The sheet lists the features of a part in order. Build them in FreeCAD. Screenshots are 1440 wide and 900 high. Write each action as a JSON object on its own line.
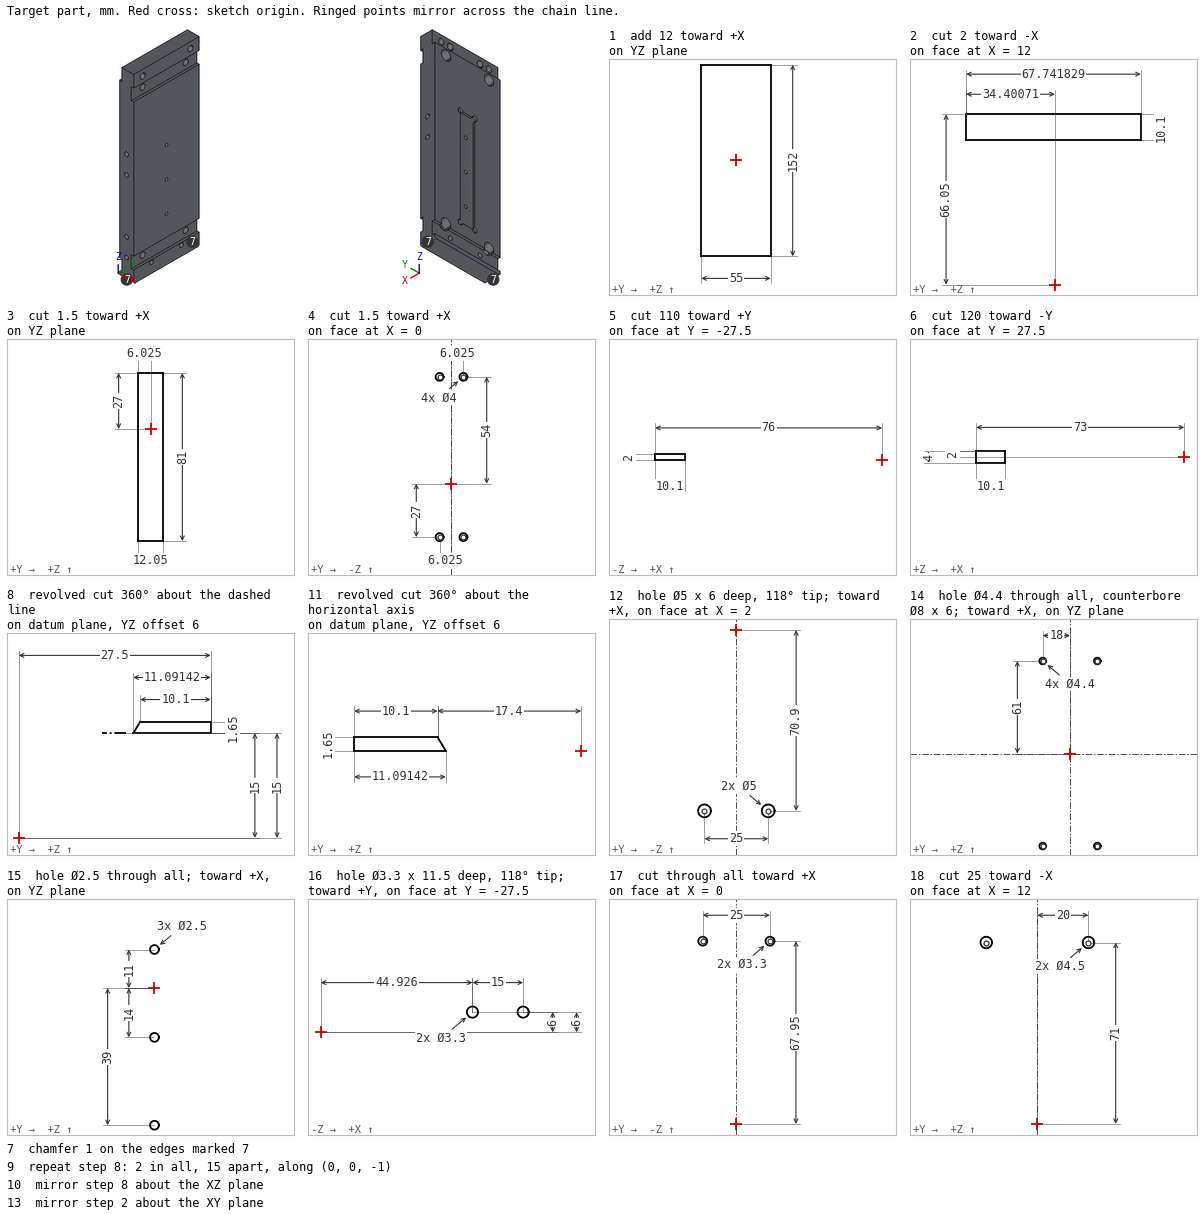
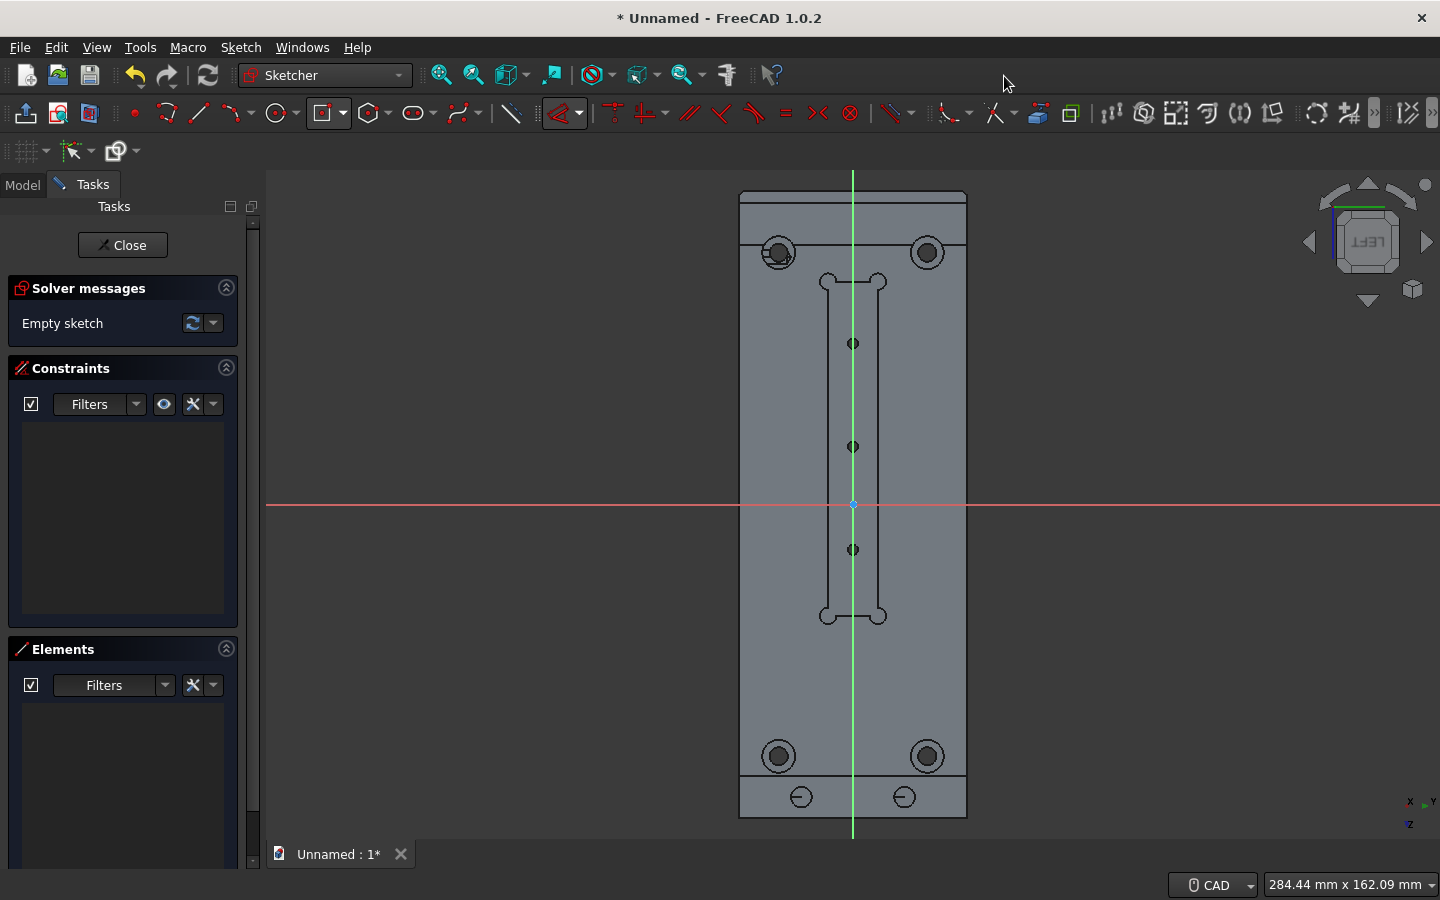
{"action": "scroll", "coordinate": [992, 198], "scroll_direction": "up", "scroll_amount": 2}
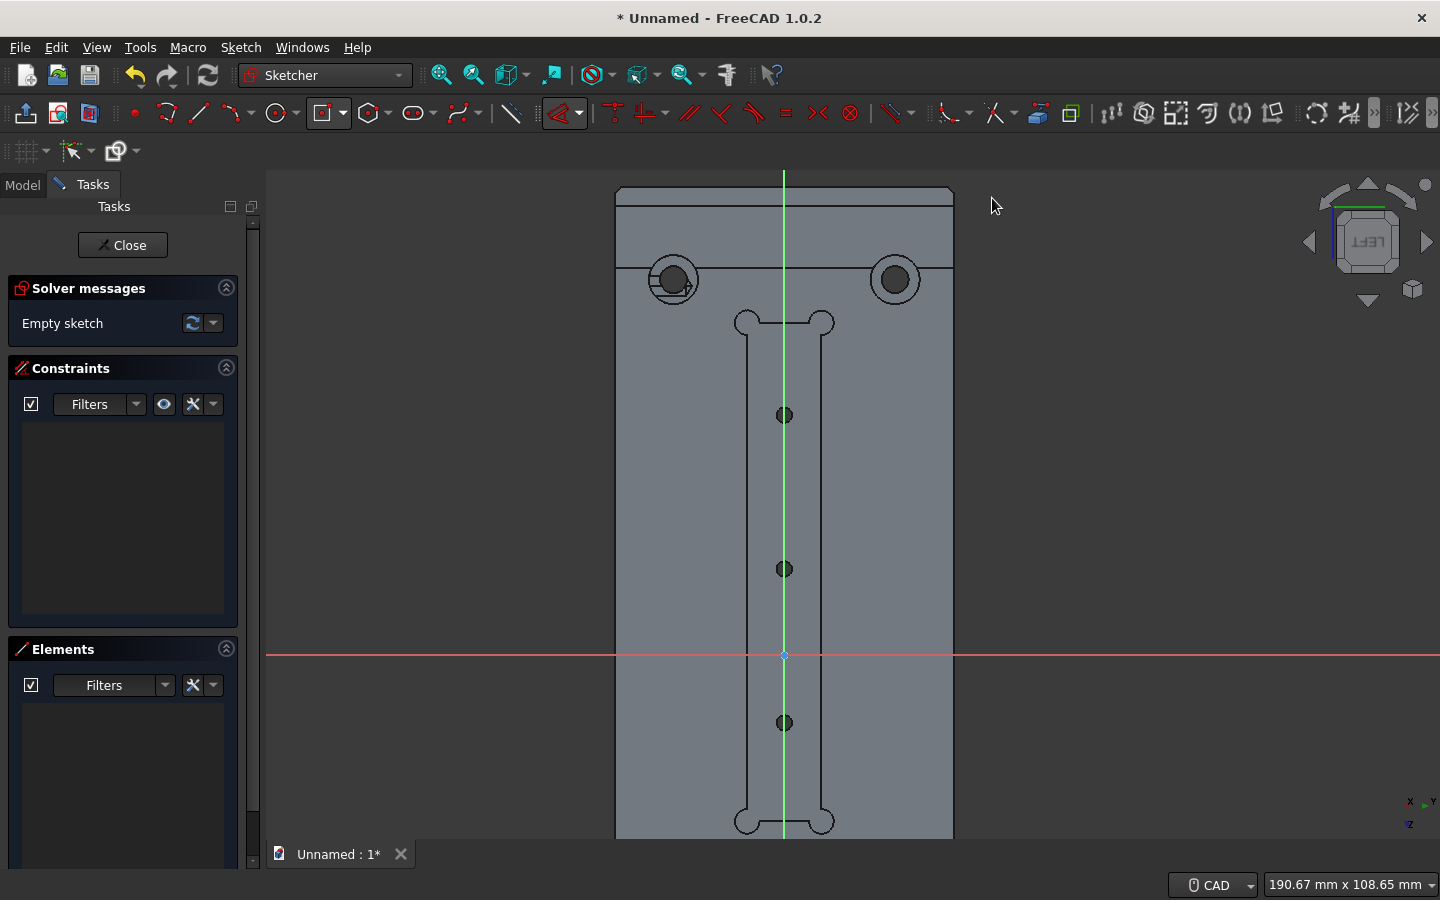
{"action": "left_click", "coordinate": [276, 114]}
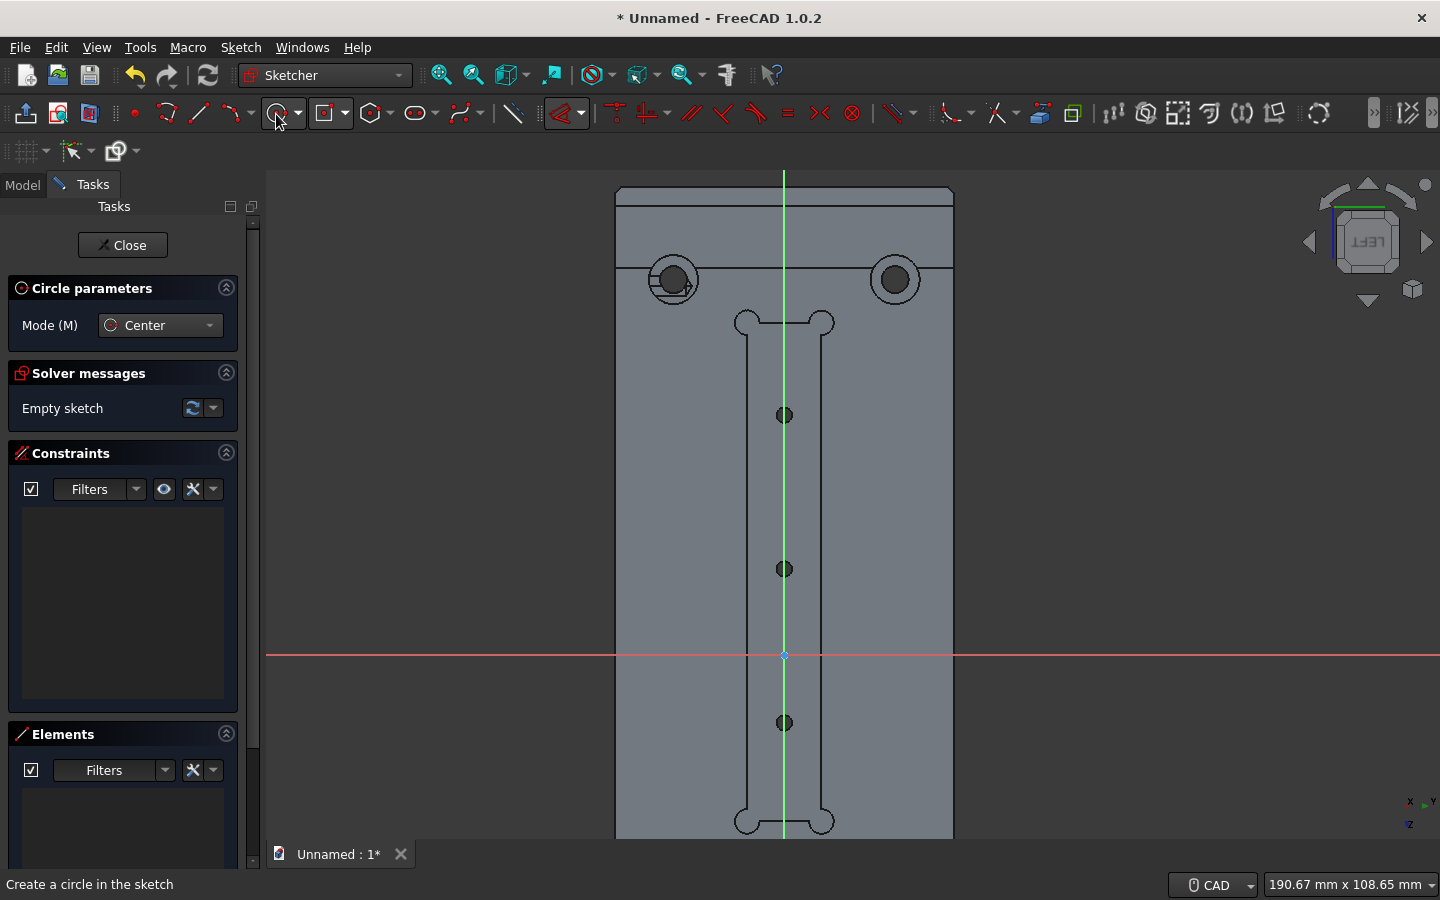
{"action": "scroll", "coordinate": [861, 237], "scroll_direction": "up", "scroll_amount": 5}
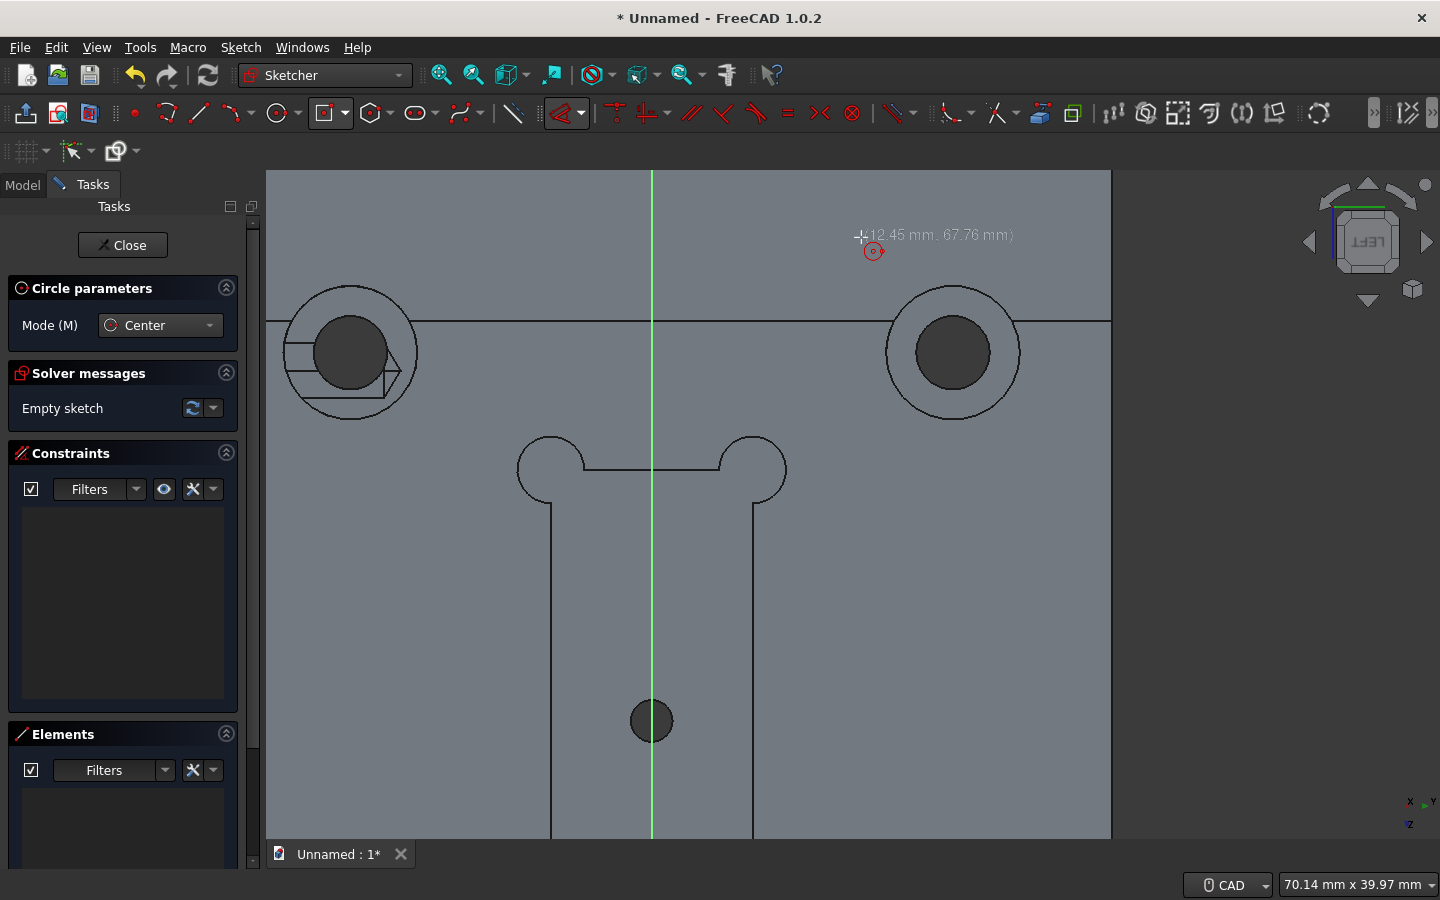
{"action": "left_click", "coordinate": [861, 236]}
{"action": "mouse_move", "coordinate": [880, 217]}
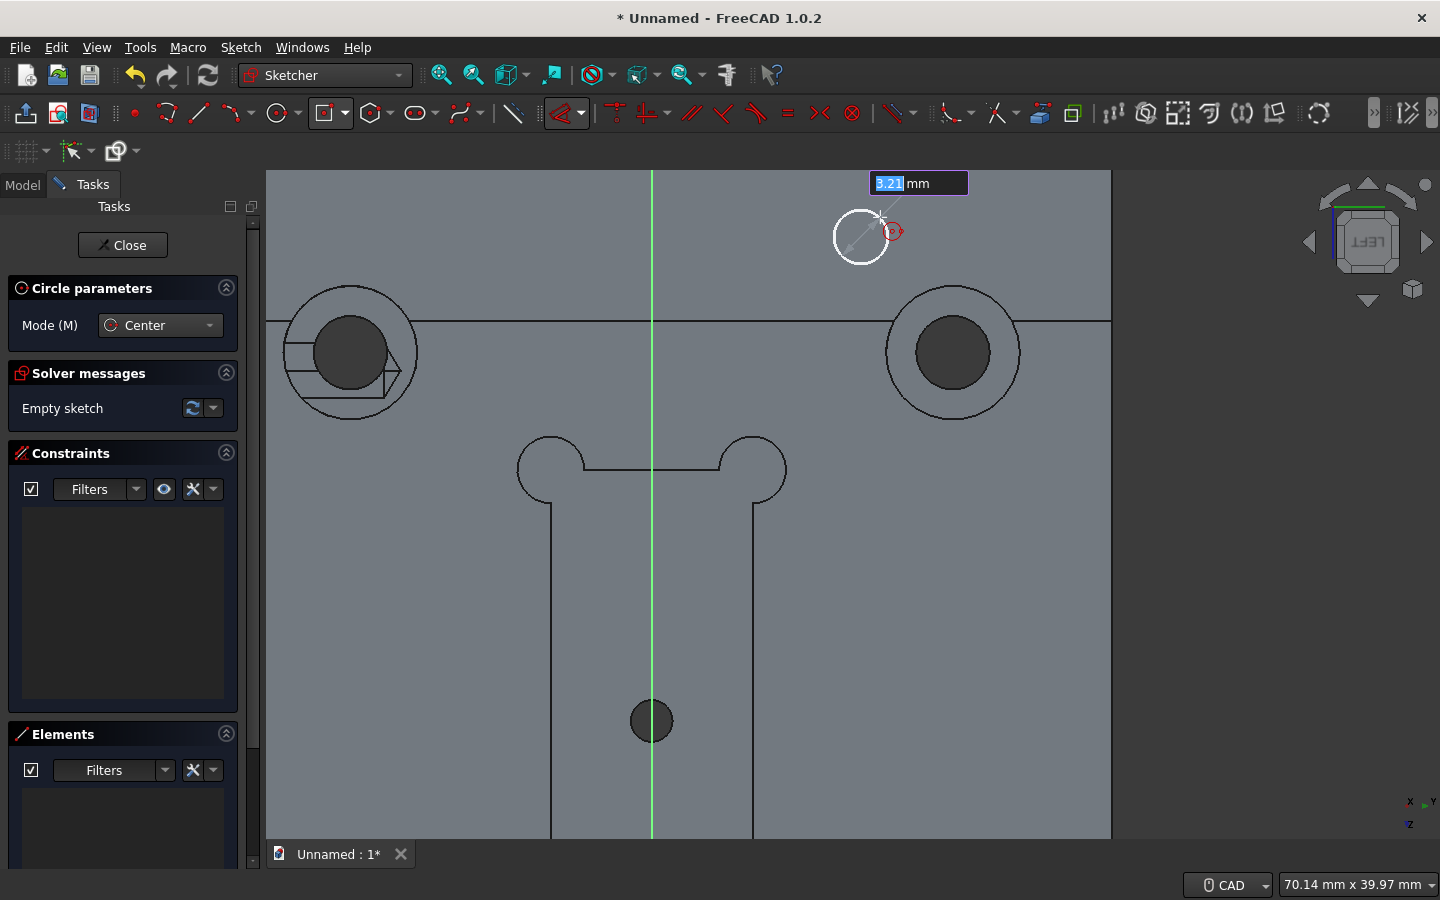
{"action": "type", "text": "3.3"}
{"action": "key", "text": "Return"}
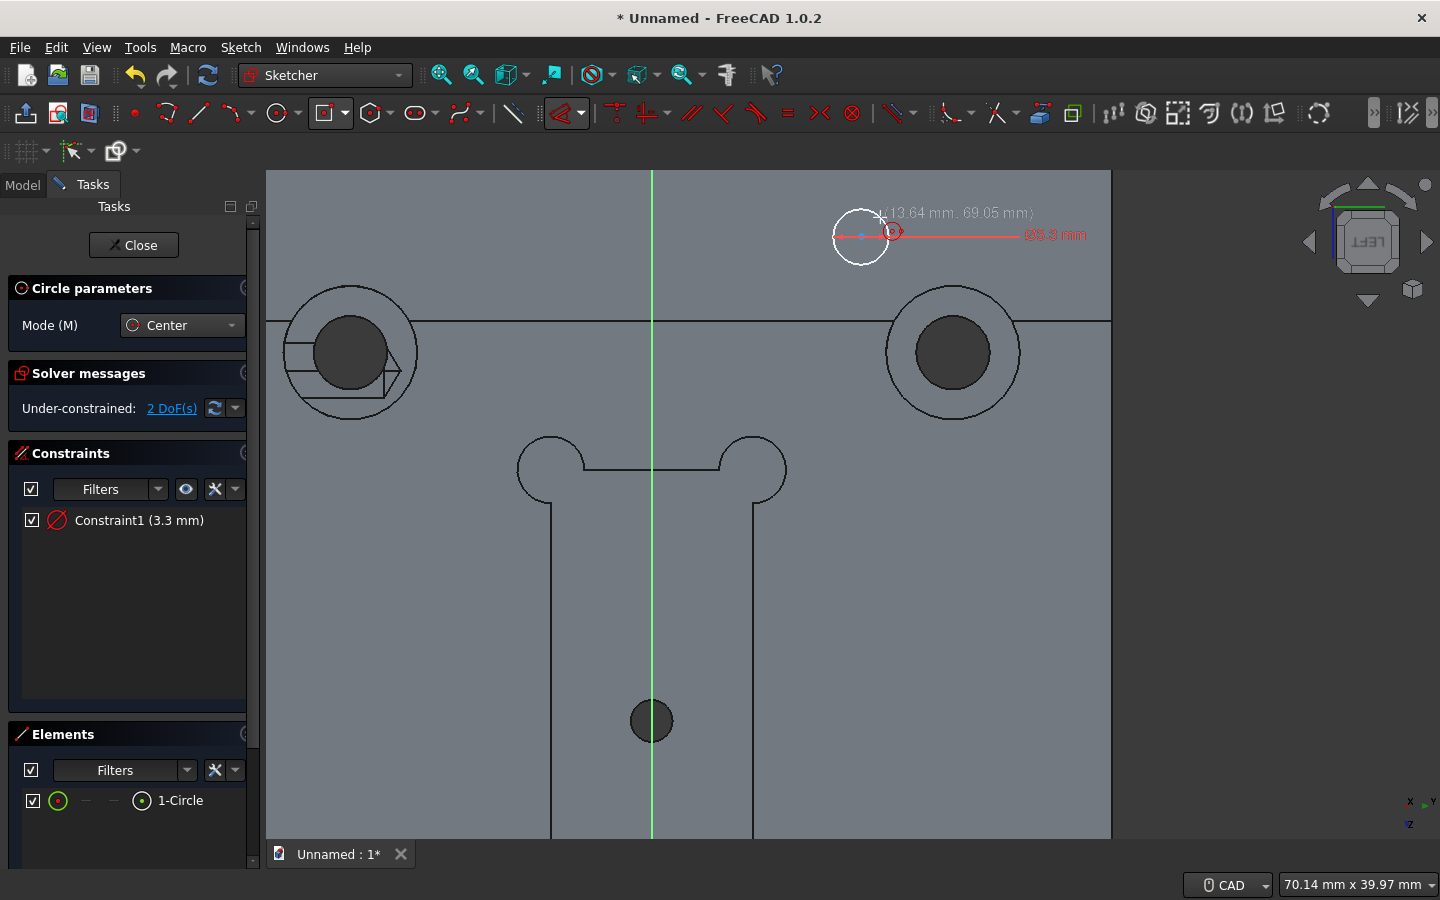
{"action": "left_click", "coordinate": [443, 236]}
{"action": "mouse_move", "coordinate": [462, 217]}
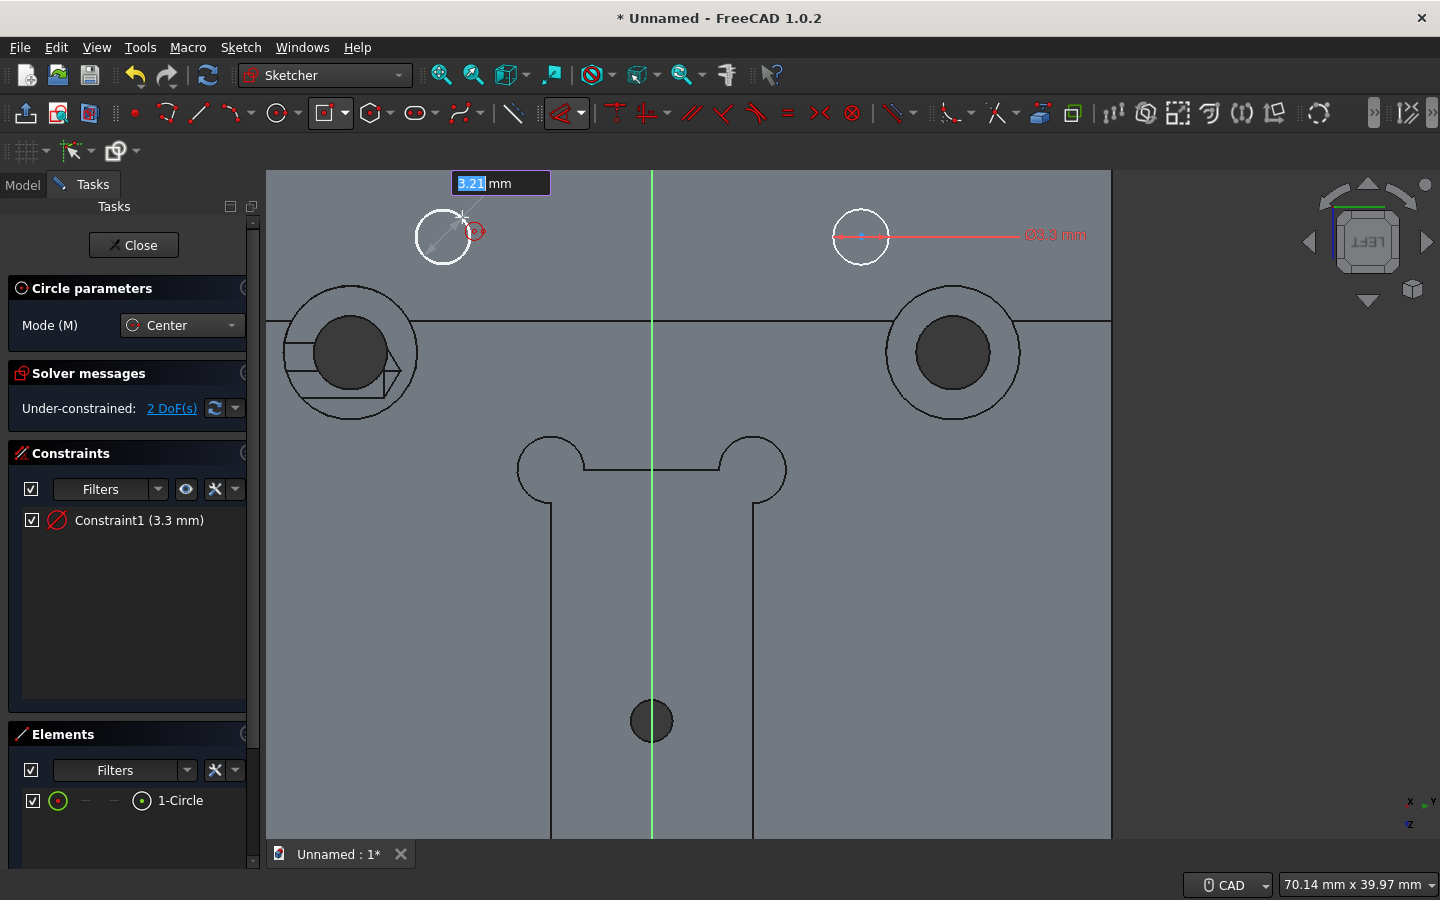
{"action": "type", "text": "3.3"}
{"action": "key", "text": "Return"}
{"action": "key", "text": "Escape"}